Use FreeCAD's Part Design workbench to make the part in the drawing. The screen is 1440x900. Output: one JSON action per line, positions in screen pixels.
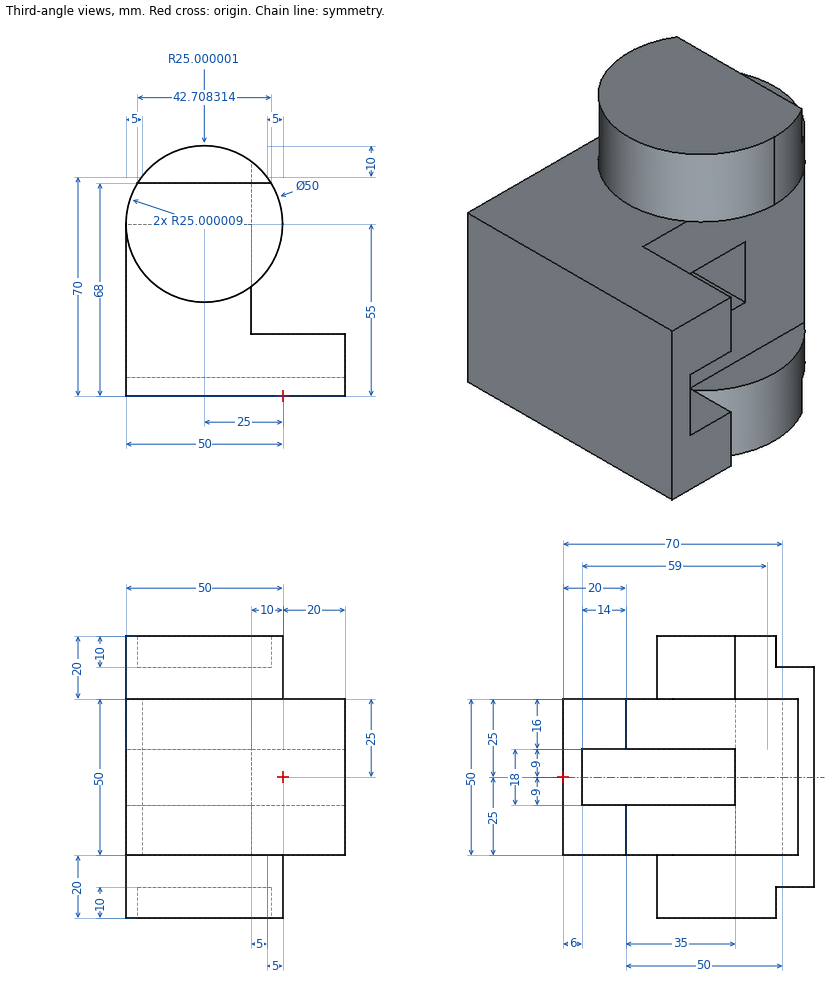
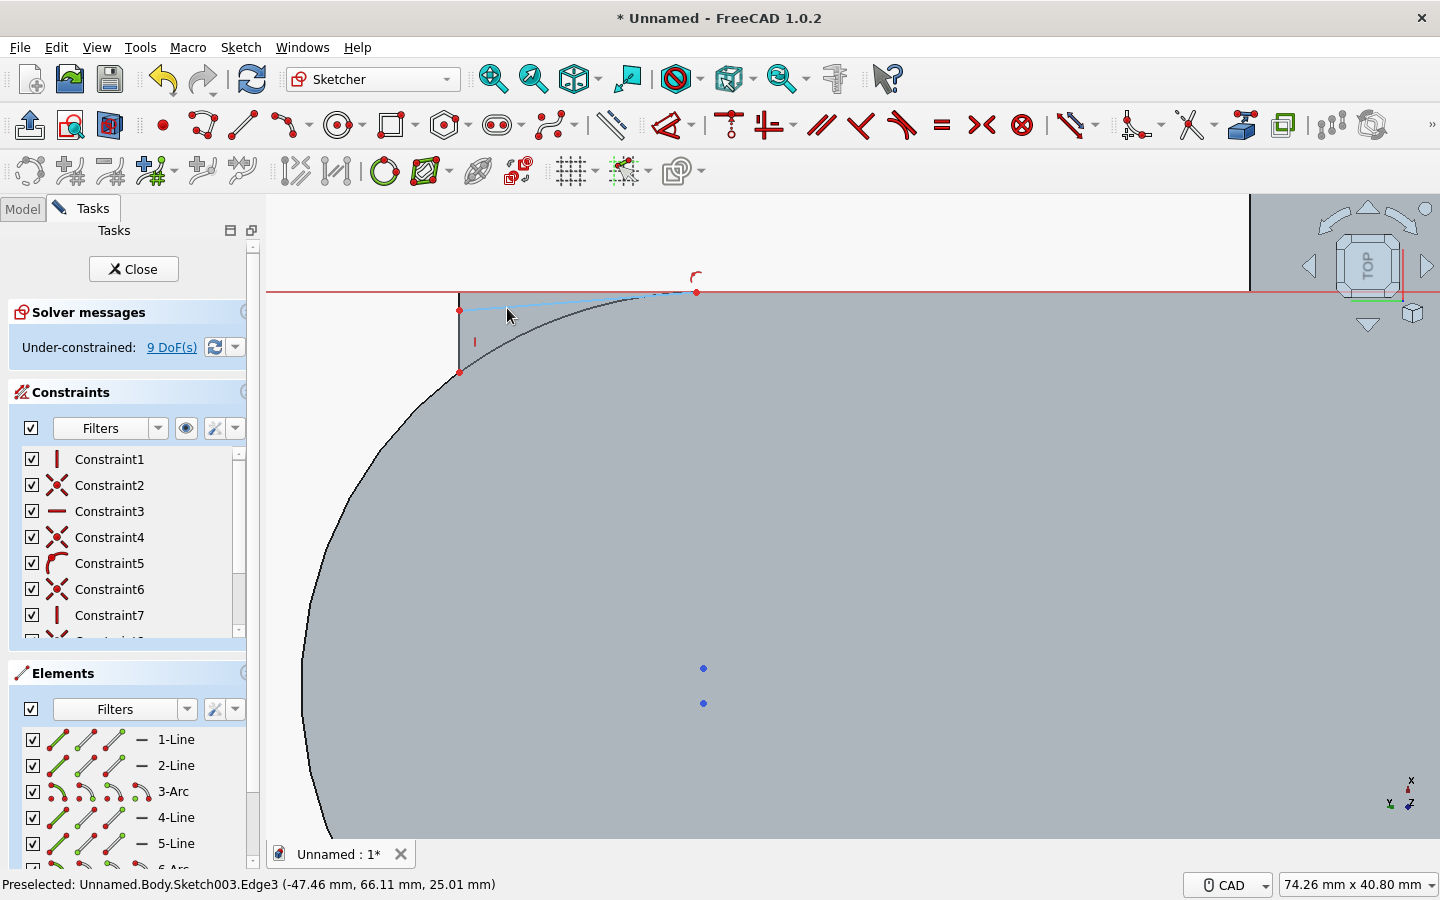
{"action": "left_click", "coordinate": [507, 307]}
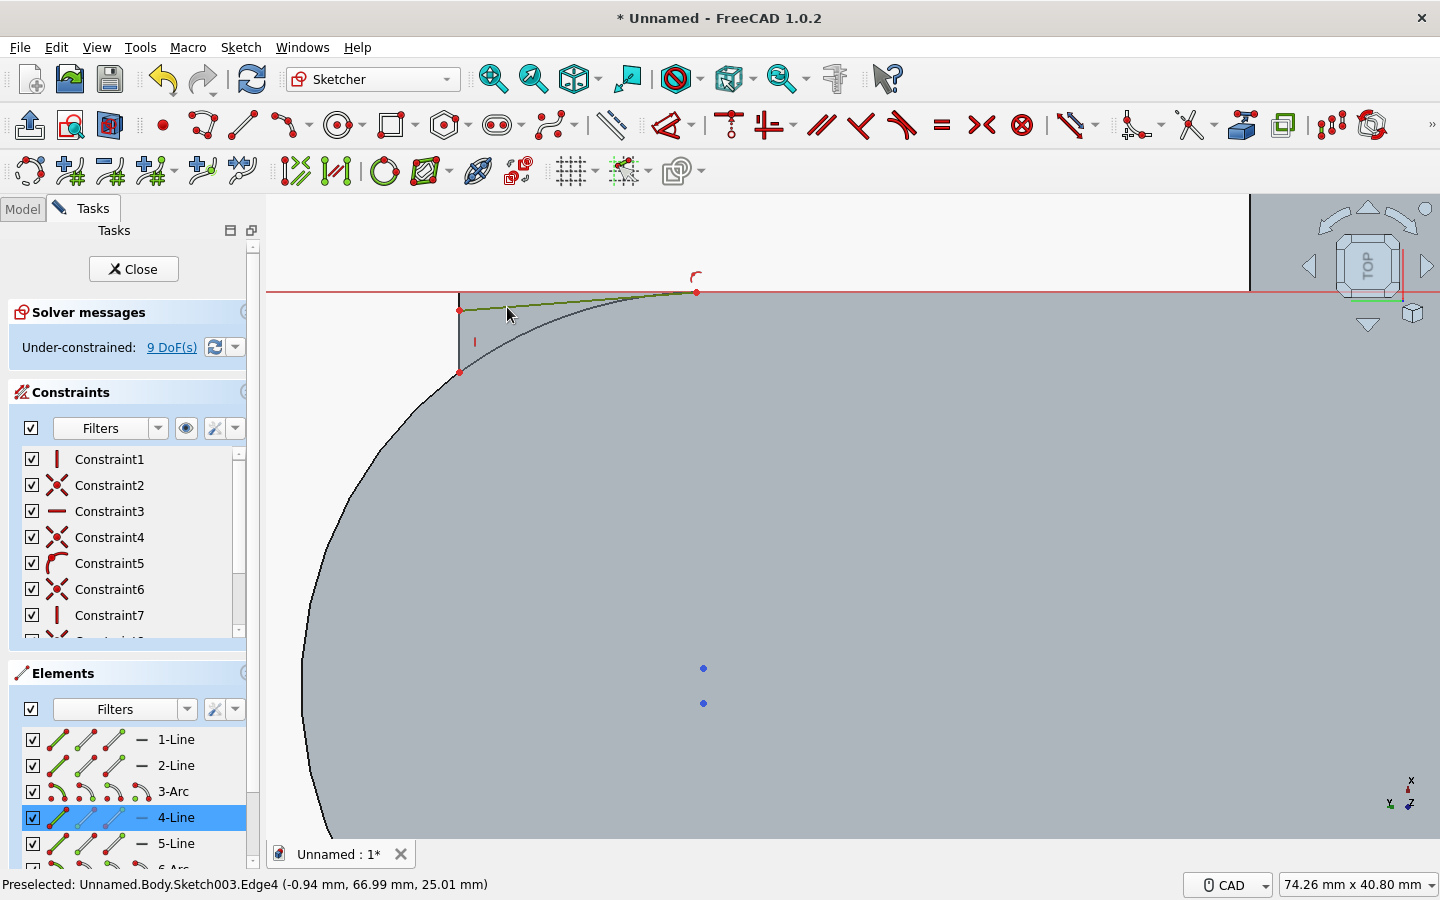
{"action": "left_click", "coordinate": [525, 333]}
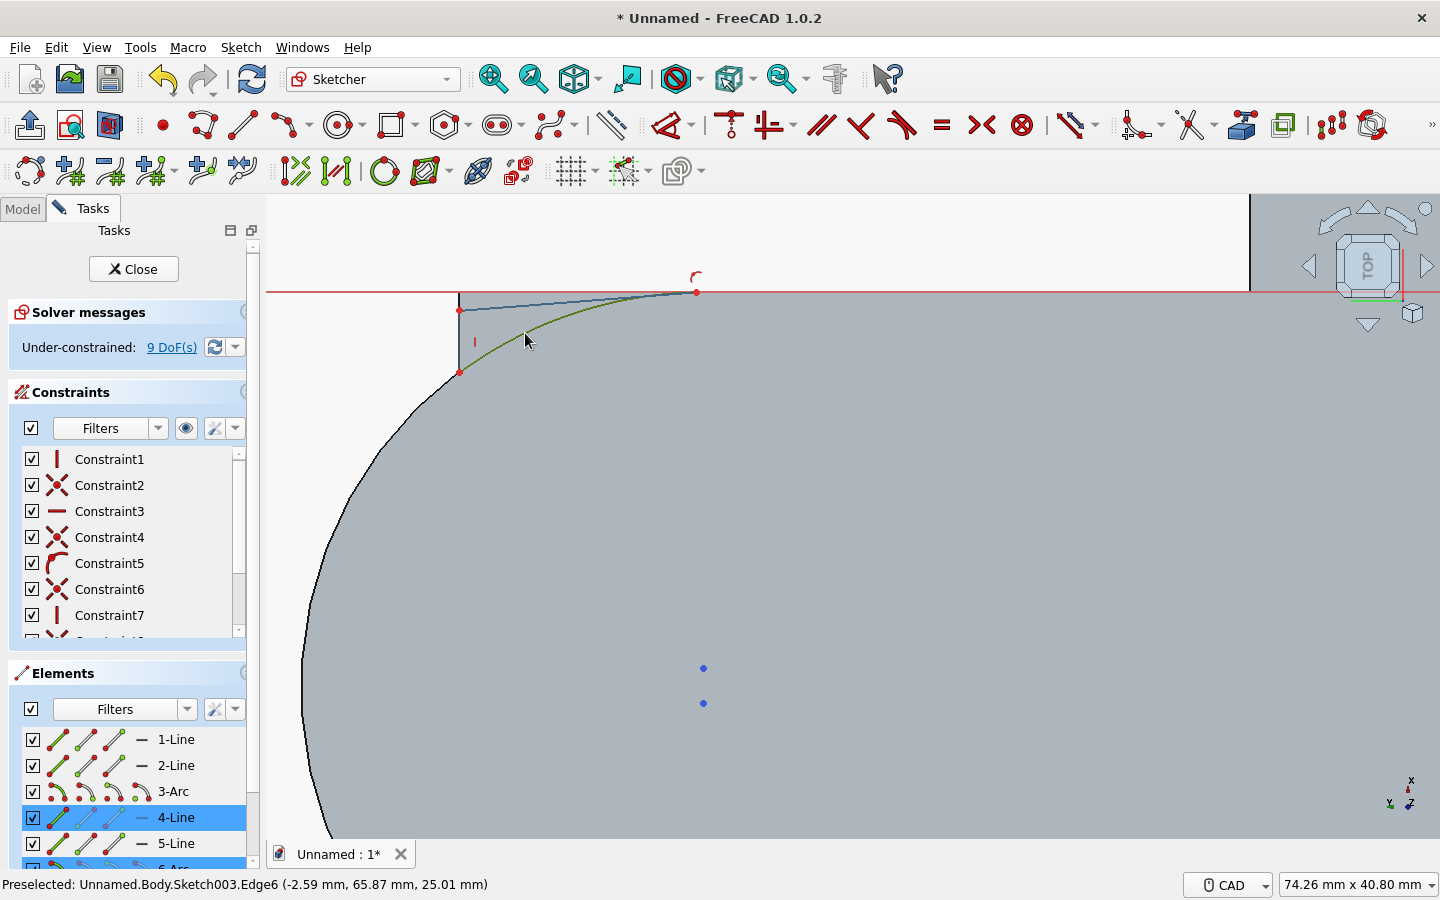
{"action": "left_click", "coordinate": [902, 126]}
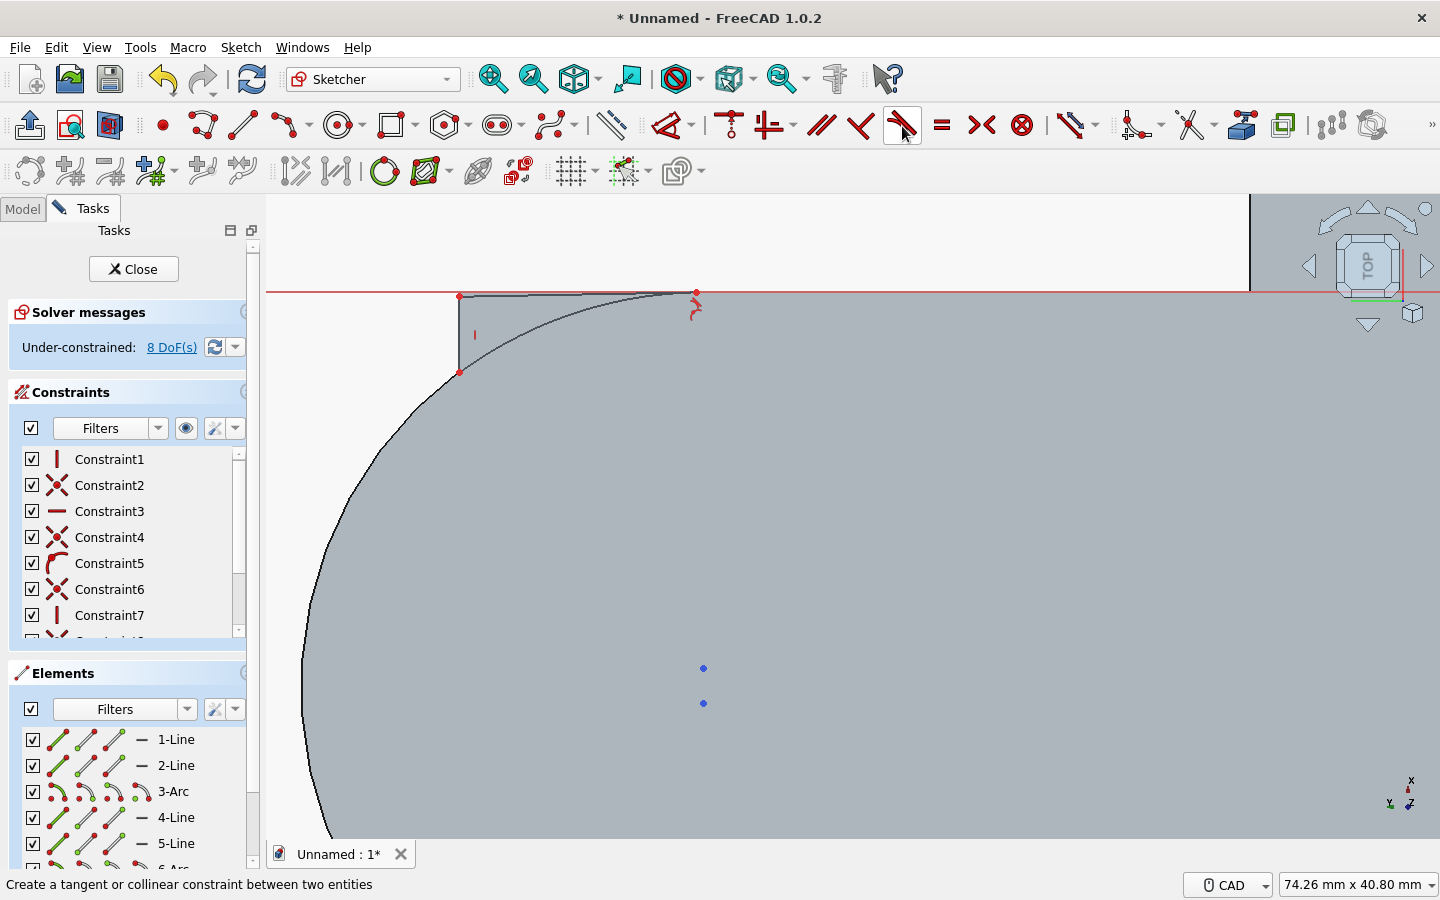
{"action": "left_click", "coordinate": [531, 295]}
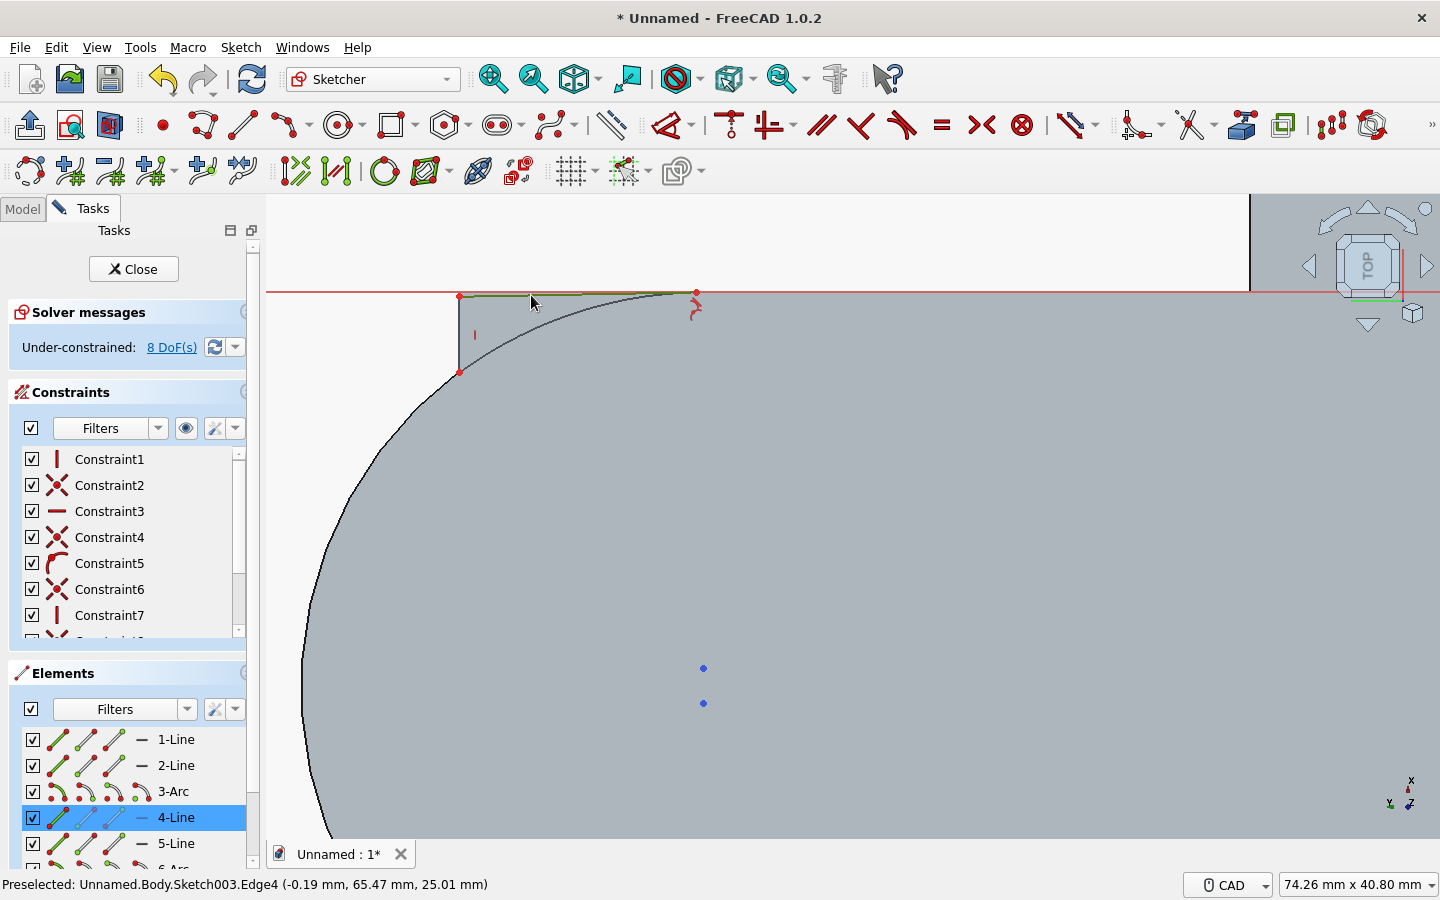
{"action": "key", "text": "h"}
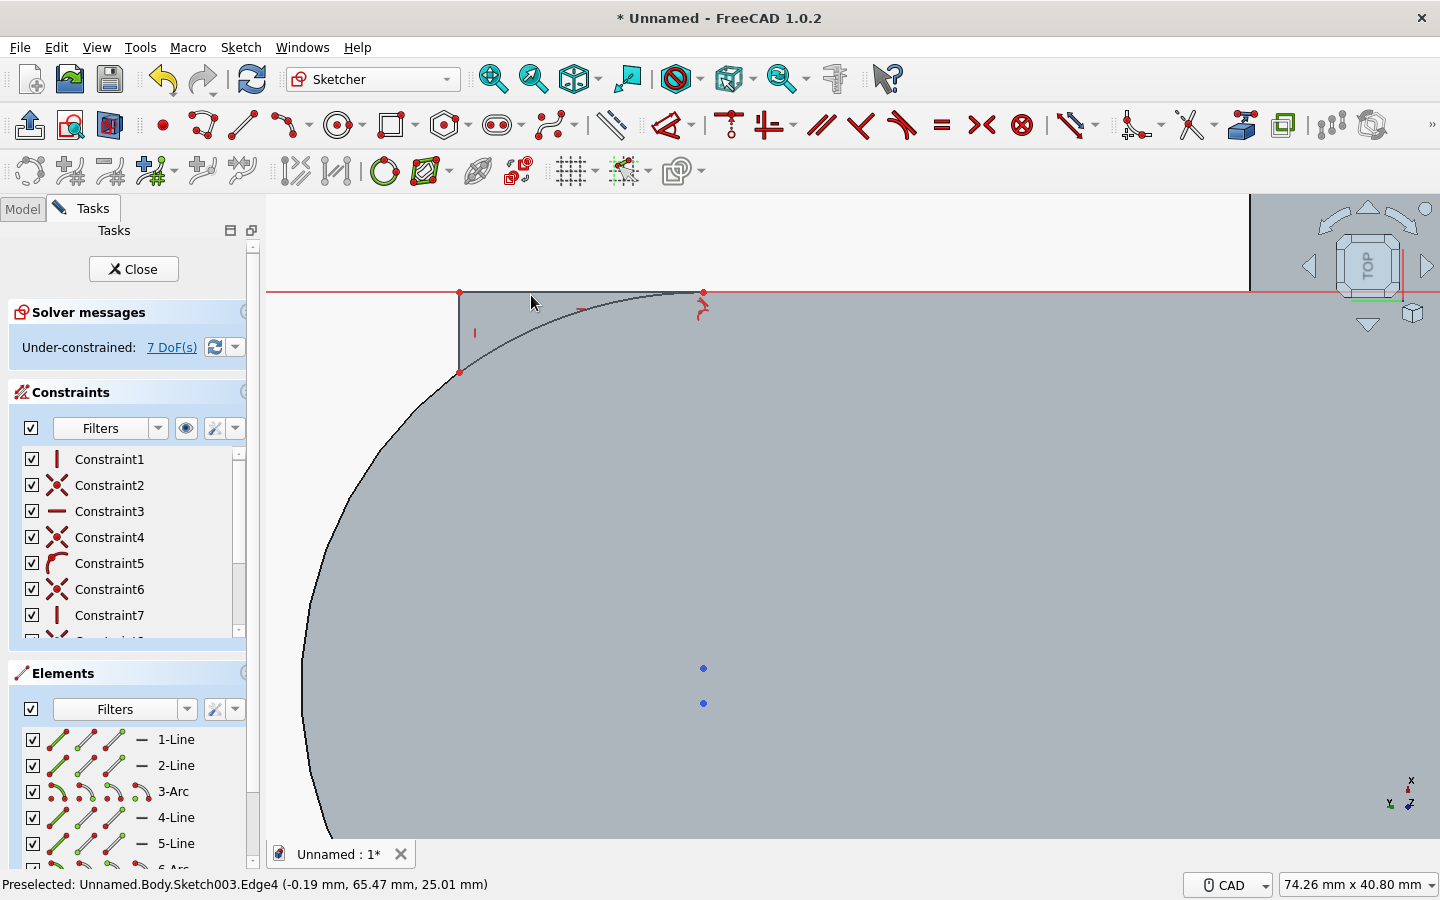
{"action": "scroll", "coordinate": [507, 308], "scroll_direction": "down", "scroll_amount": 3}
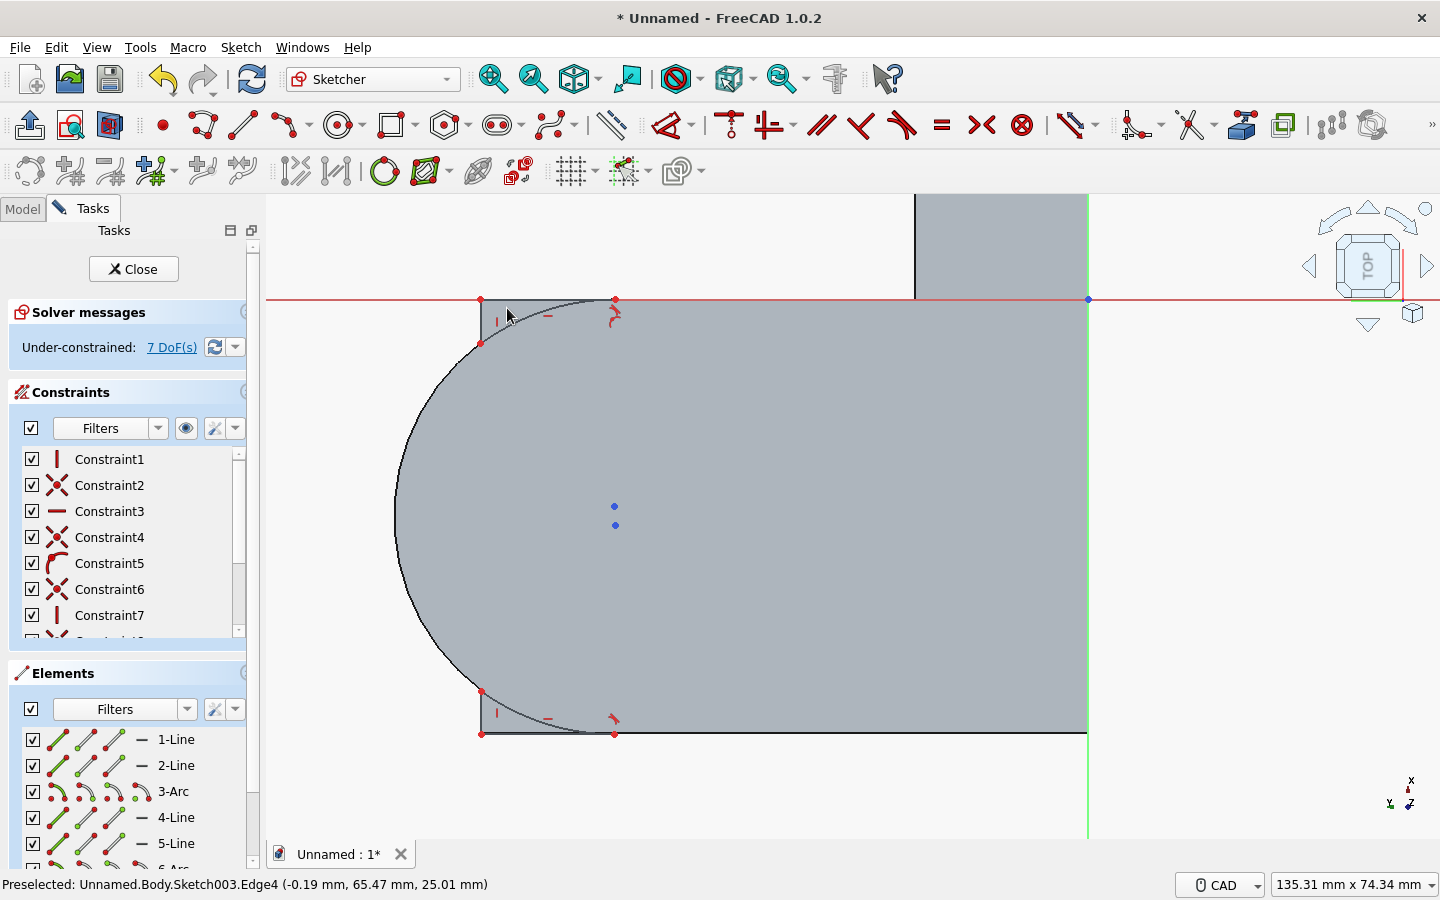
{"action": "left_click", "coordinate": [518, 713]}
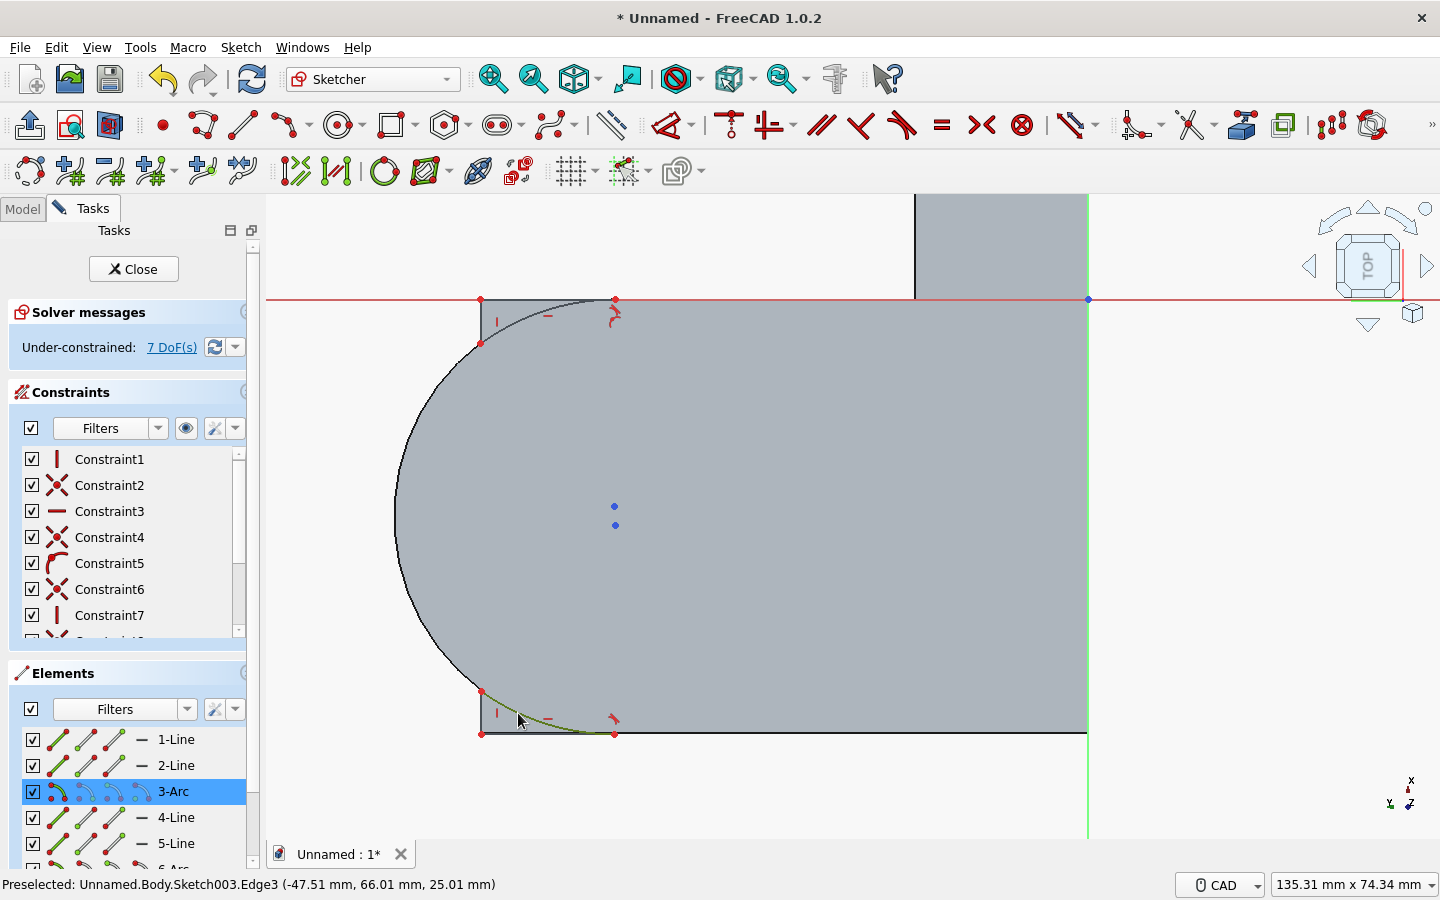
{"action": "left_click", "coordinate": [518, 322]}